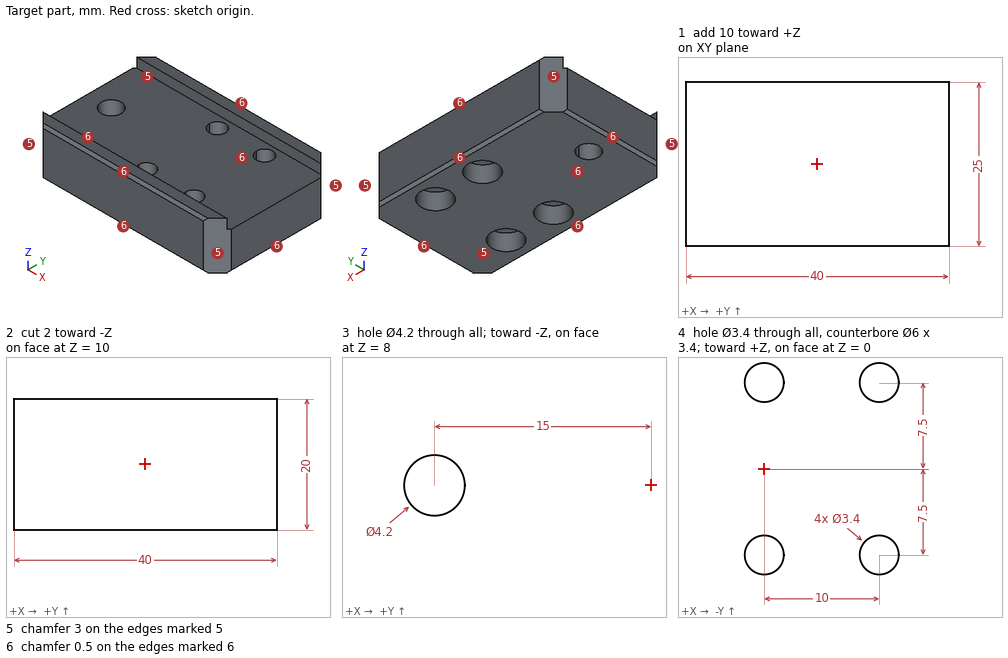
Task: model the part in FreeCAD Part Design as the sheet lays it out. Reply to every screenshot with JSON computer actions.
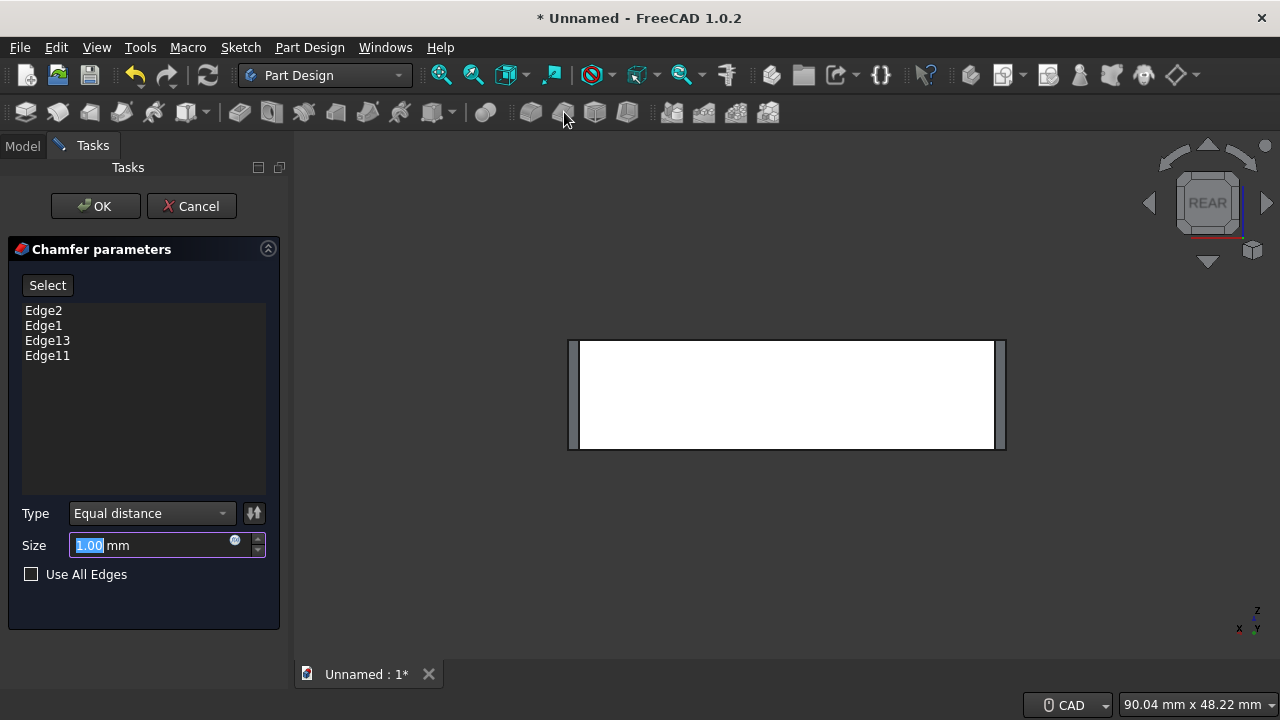
{"action": "type", "text": "3"}
{"action": "key", "text": "Tab"}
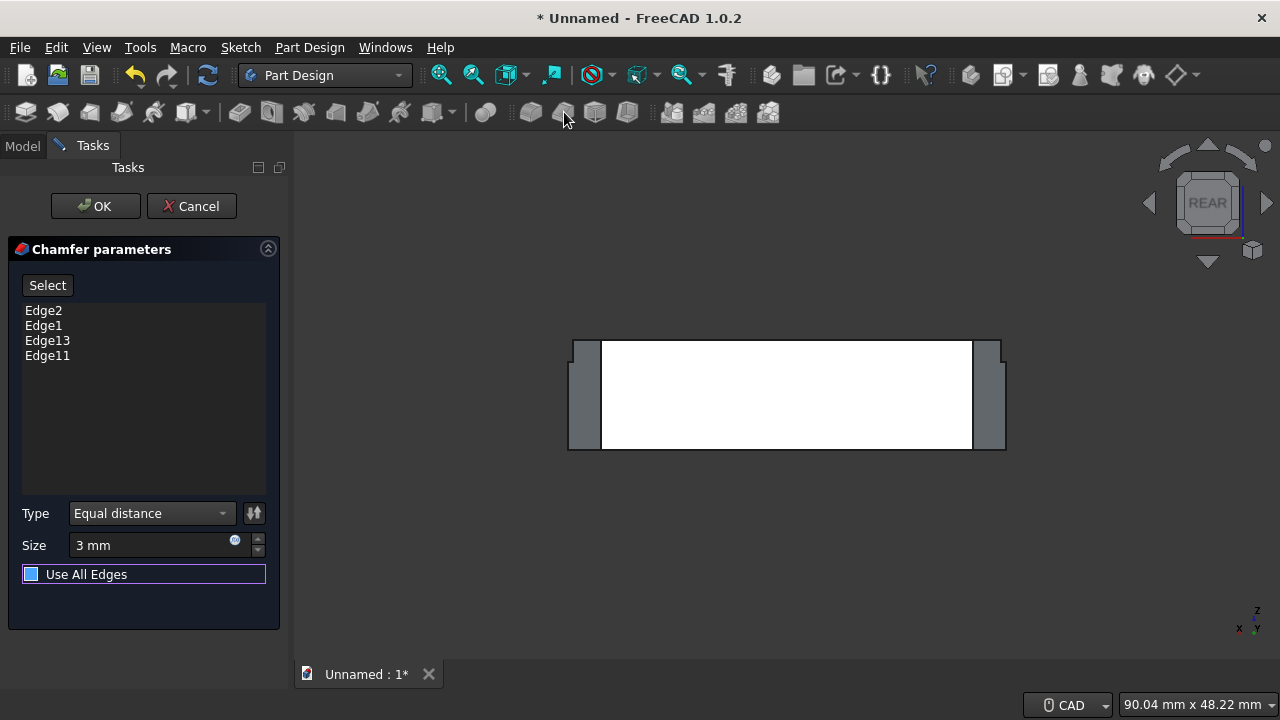
{"action": "left_click", "coordinate": [96, 206]}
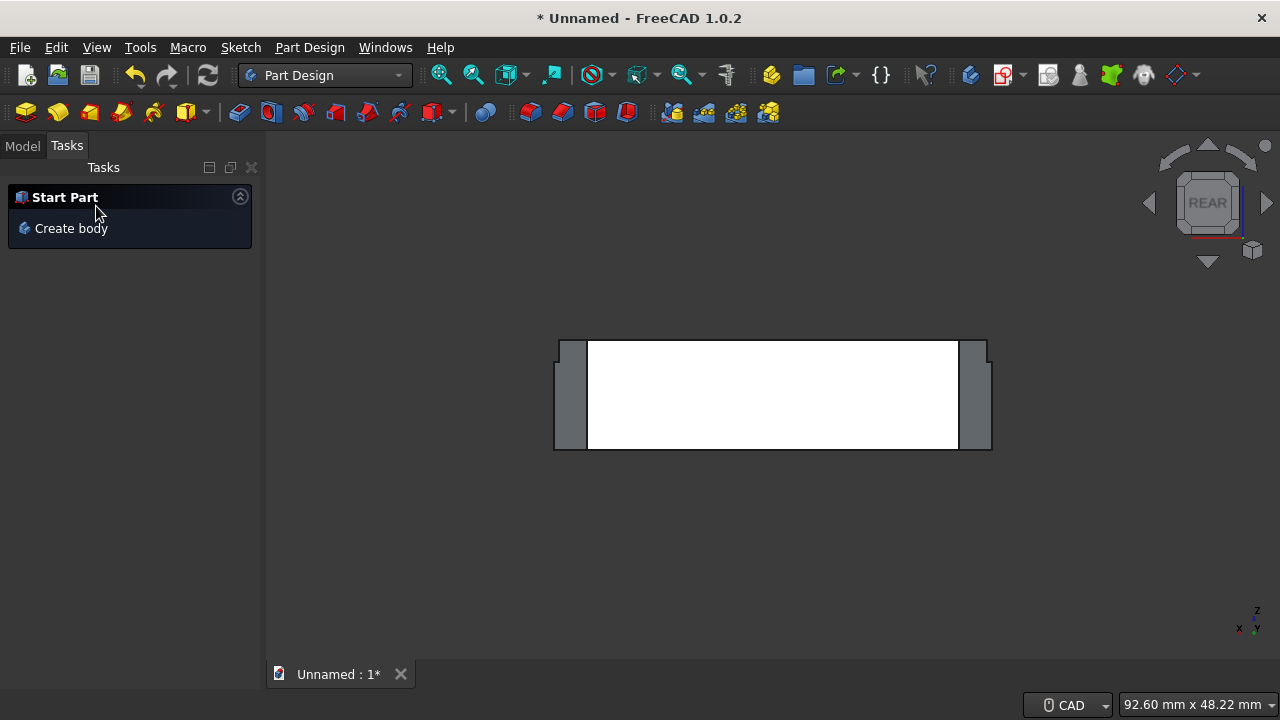
{"action": "left_click", "coordinate": [442, 76]}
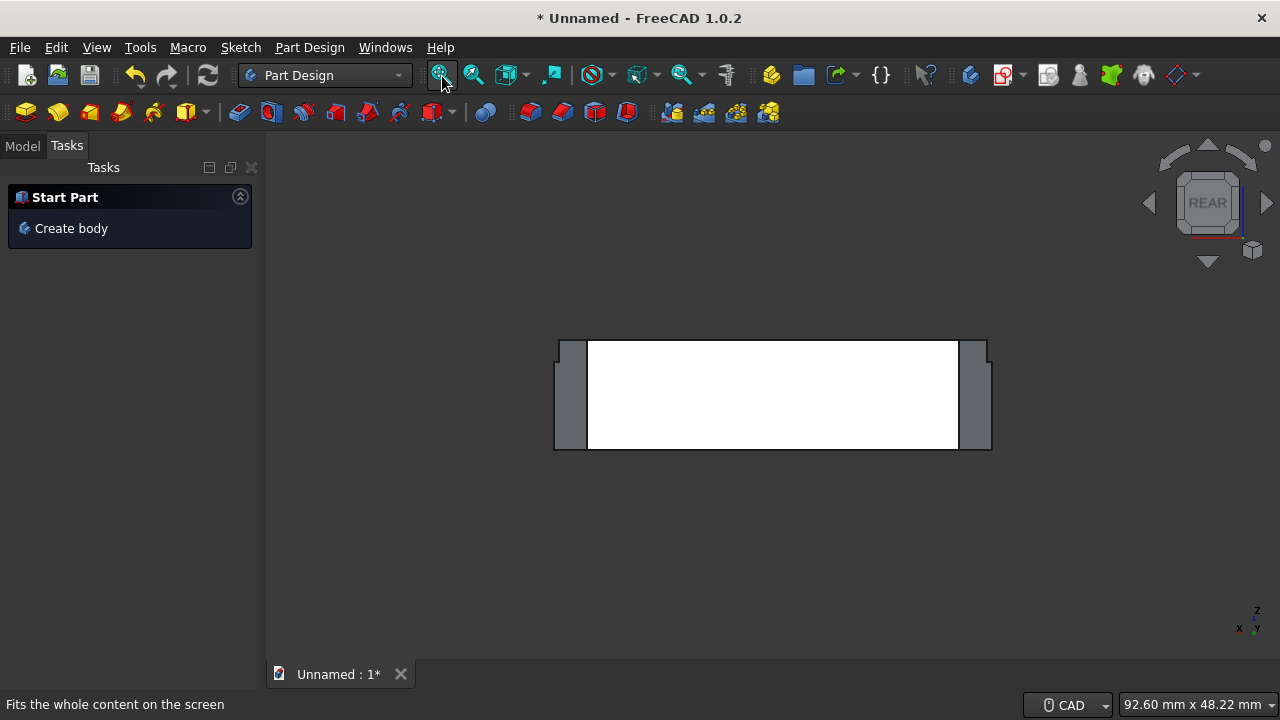
{"action": "left_click", "coordinate": [773, 449]}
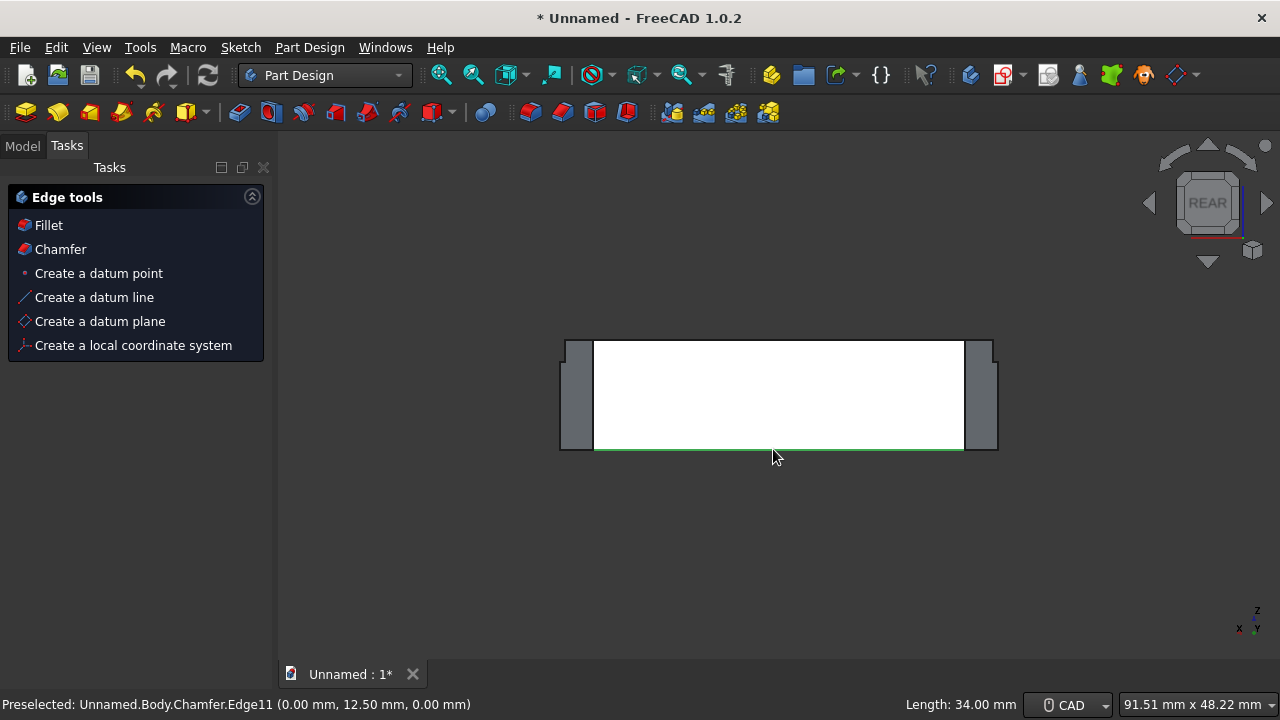
{"action": "left_click", "coordinate": [779, 339], "text": "ctrl"}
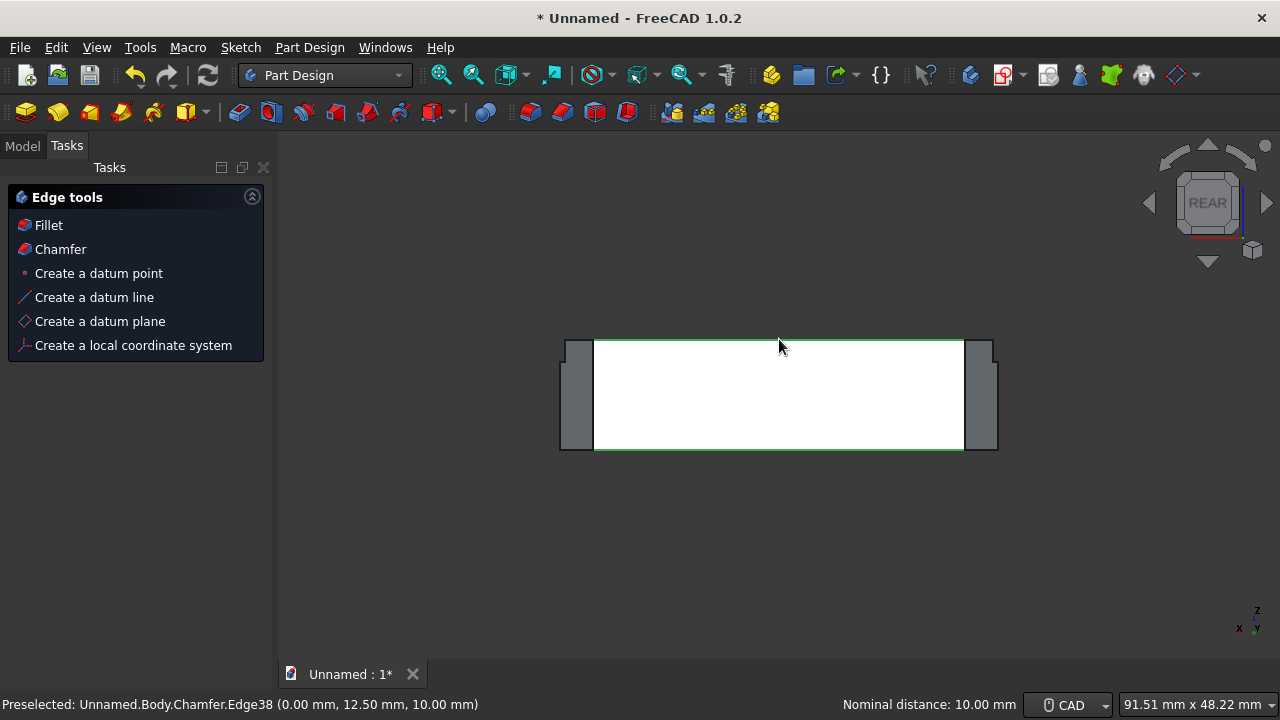
{"action": "key", "text": "0"}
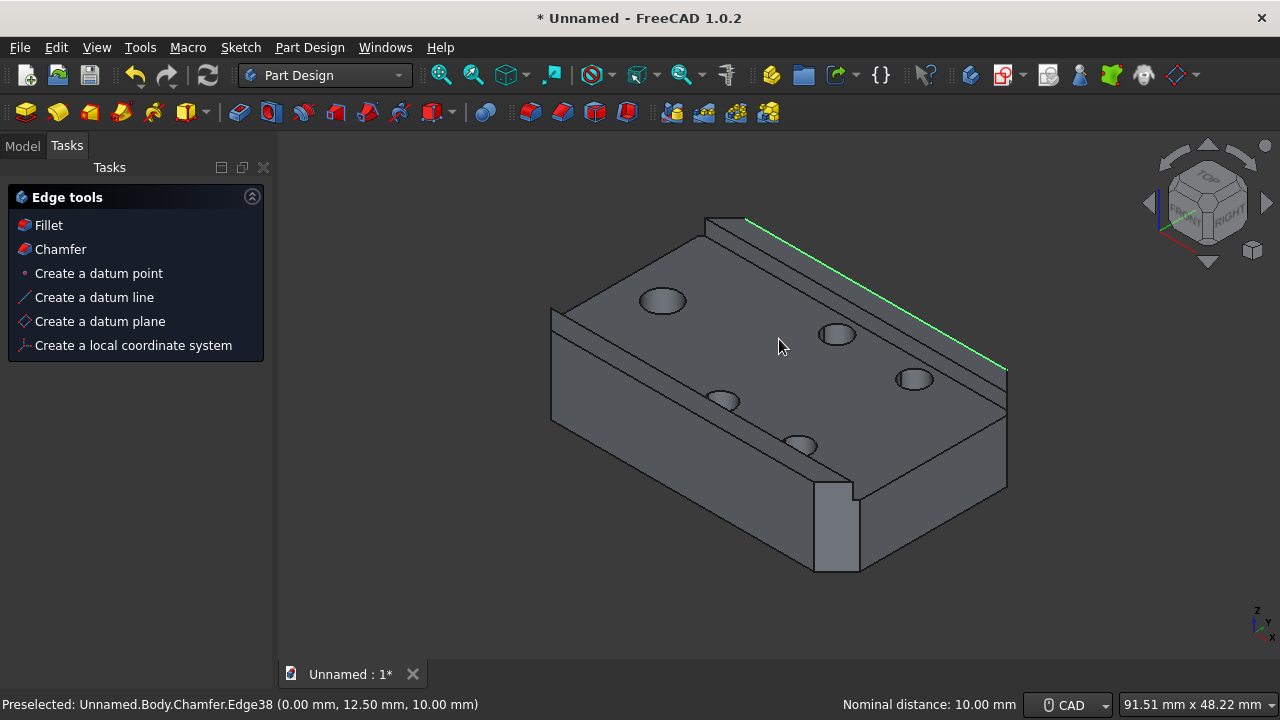
{"action": "left_click", "coordinate": [682, 405], "text": "ctrl"}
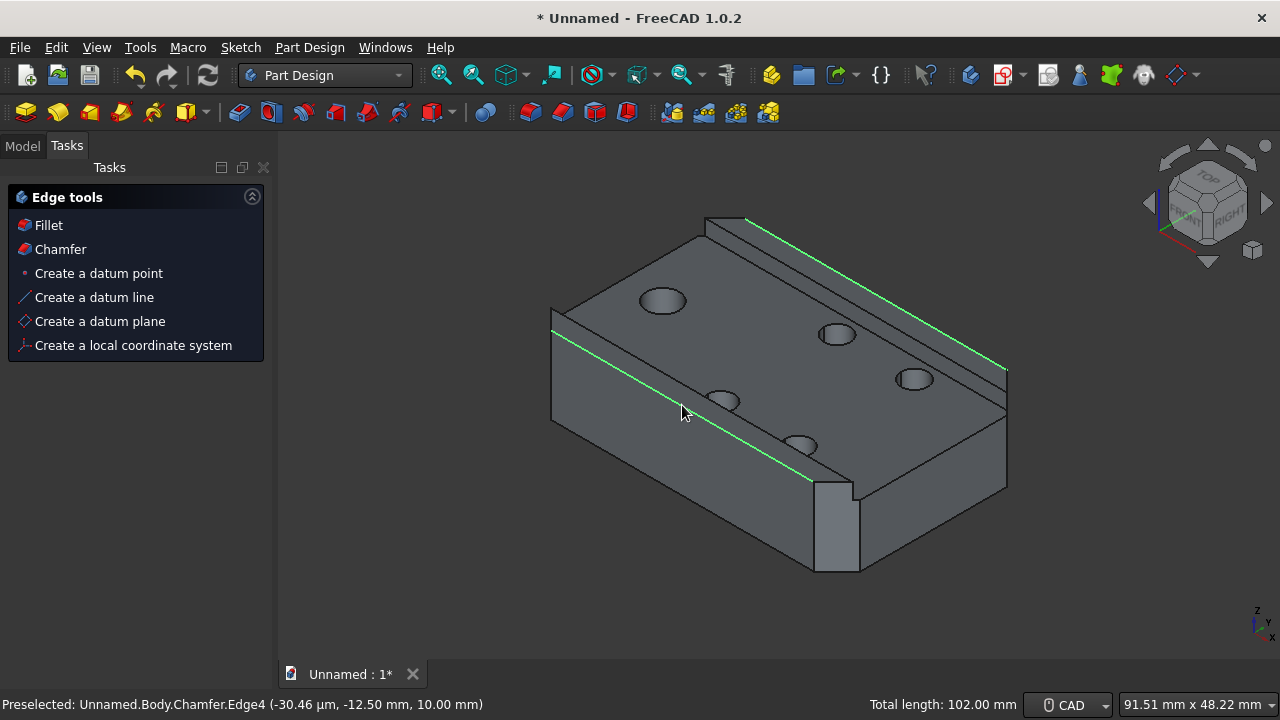
{"action": "key", "text": "2"}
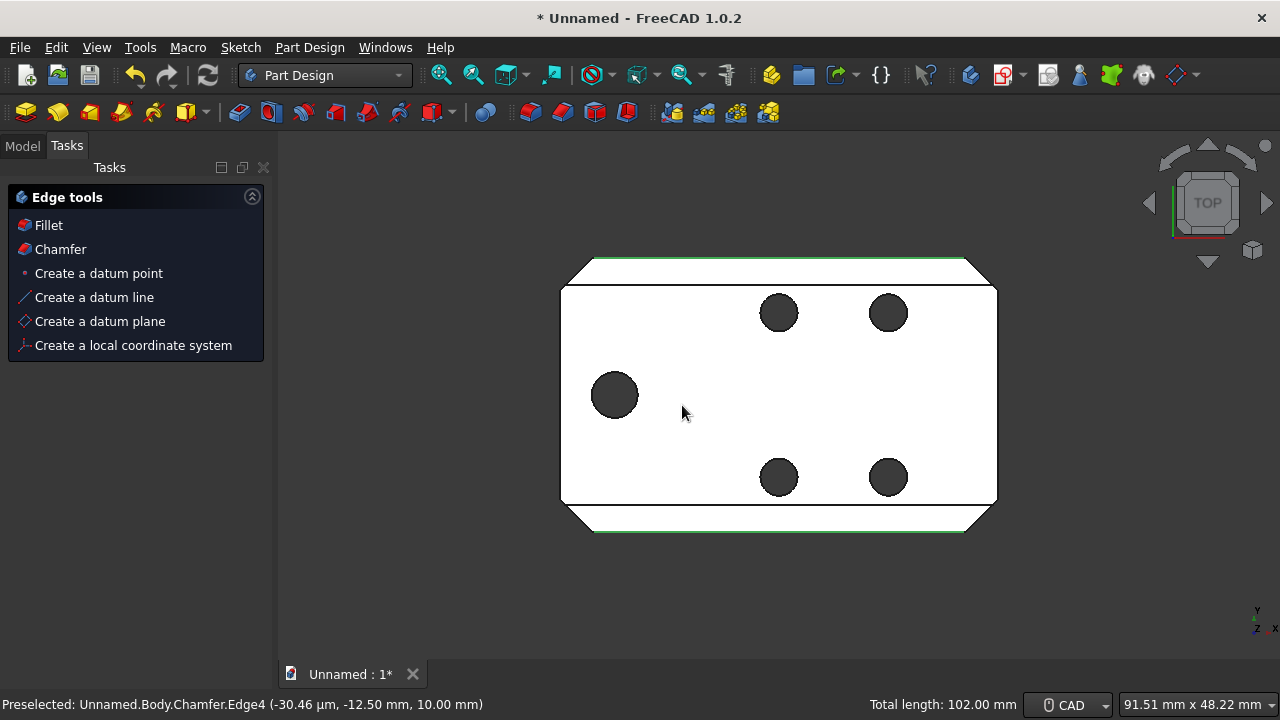
{"action": "key", "text": "1"}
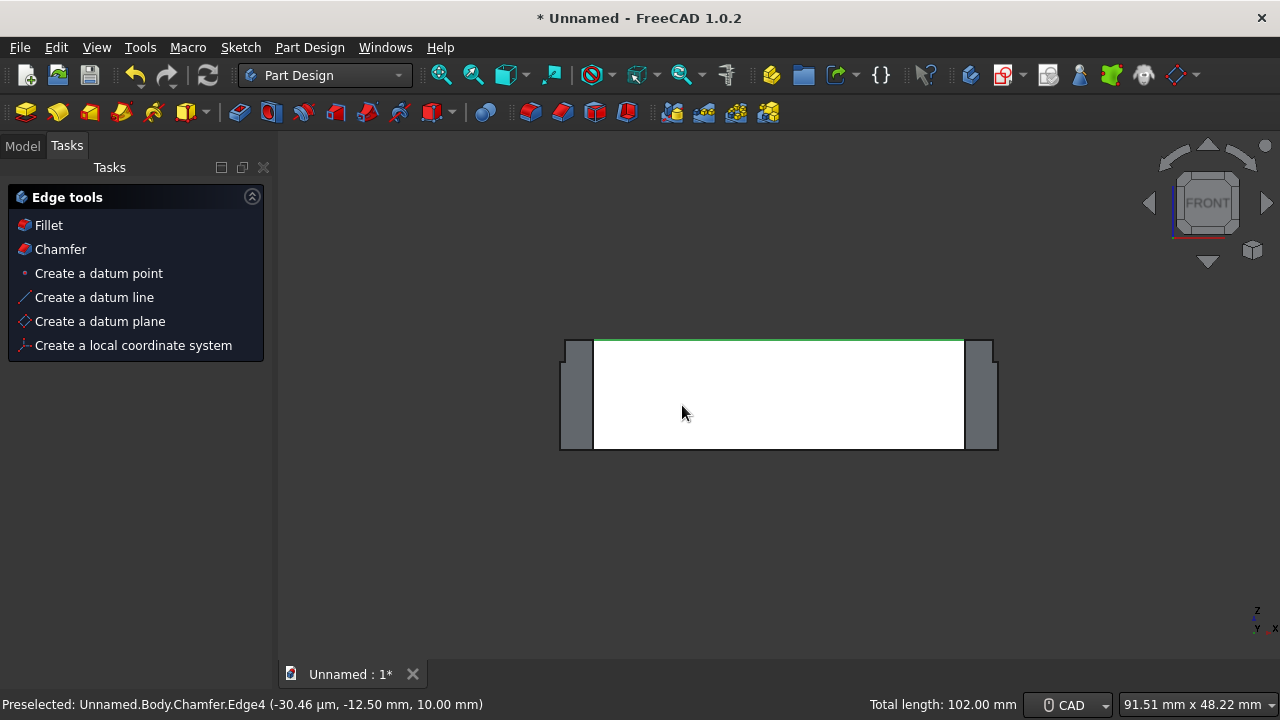
{"action": "left_click", "coordinate": [442, 76]}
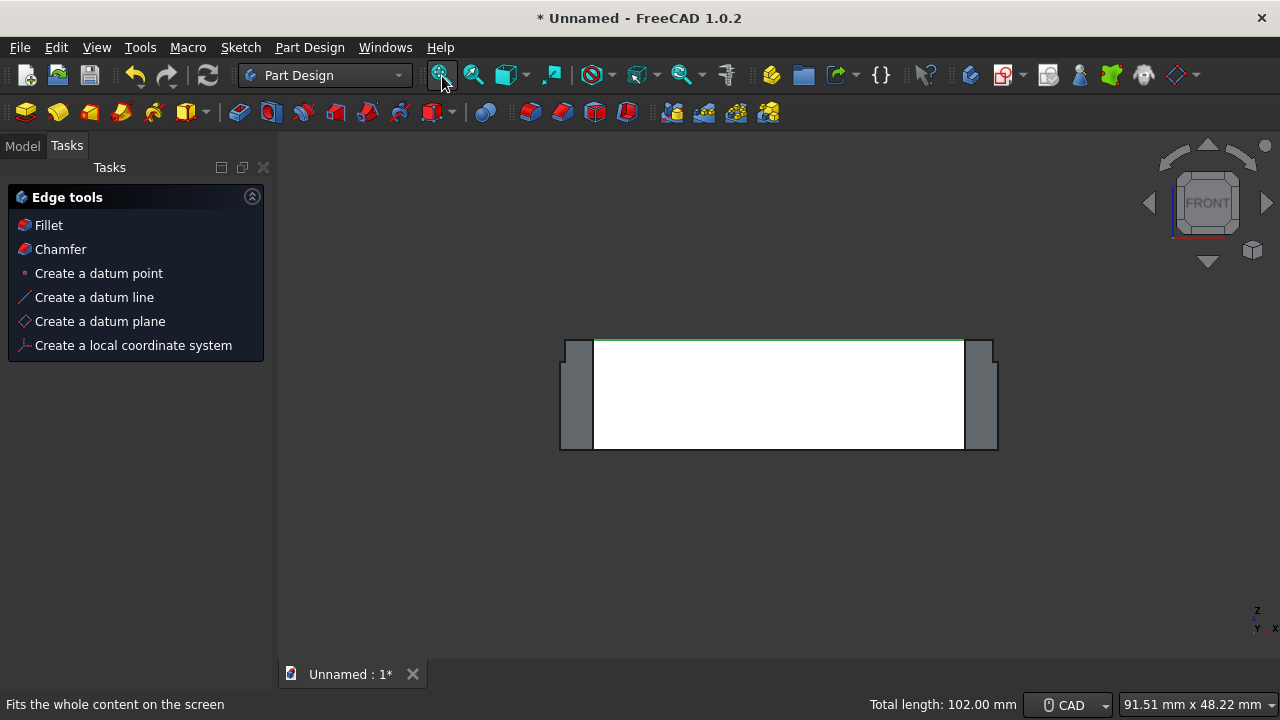
{"action": "left_click", "coordinate": [779, 449], "text": "ctrl"}